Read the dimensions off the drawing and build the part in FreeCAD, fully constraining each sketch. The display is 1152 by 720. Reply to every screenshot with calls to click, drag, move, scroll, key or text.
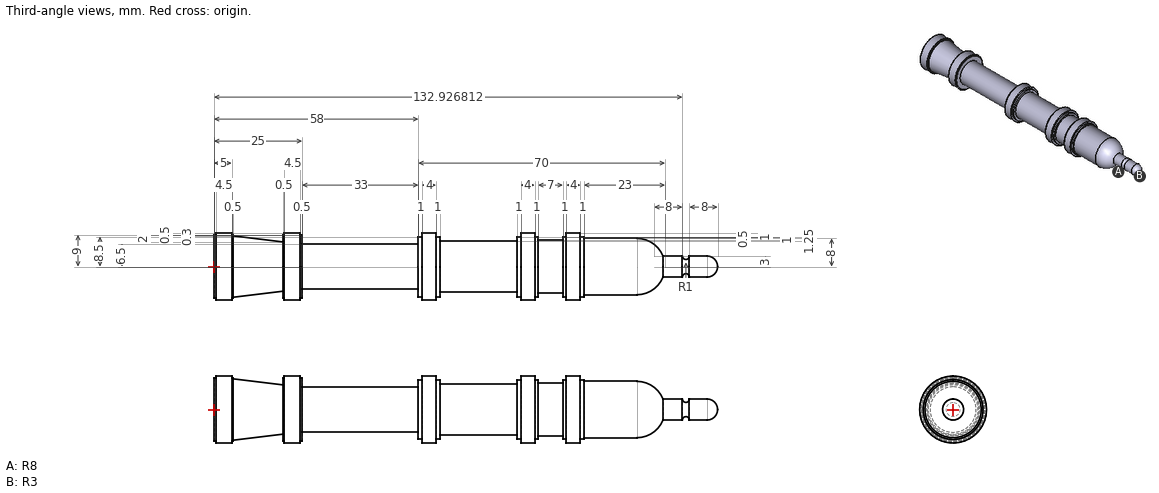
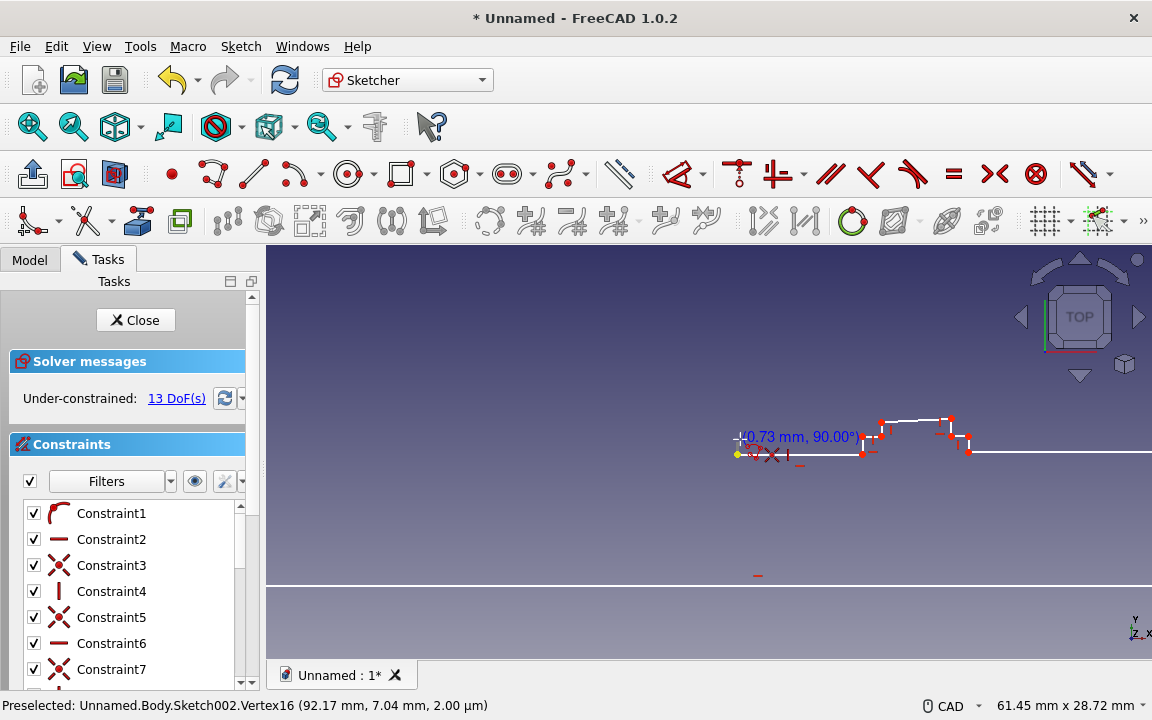
click(738, 436)
click(722, 436)
click(722, 419)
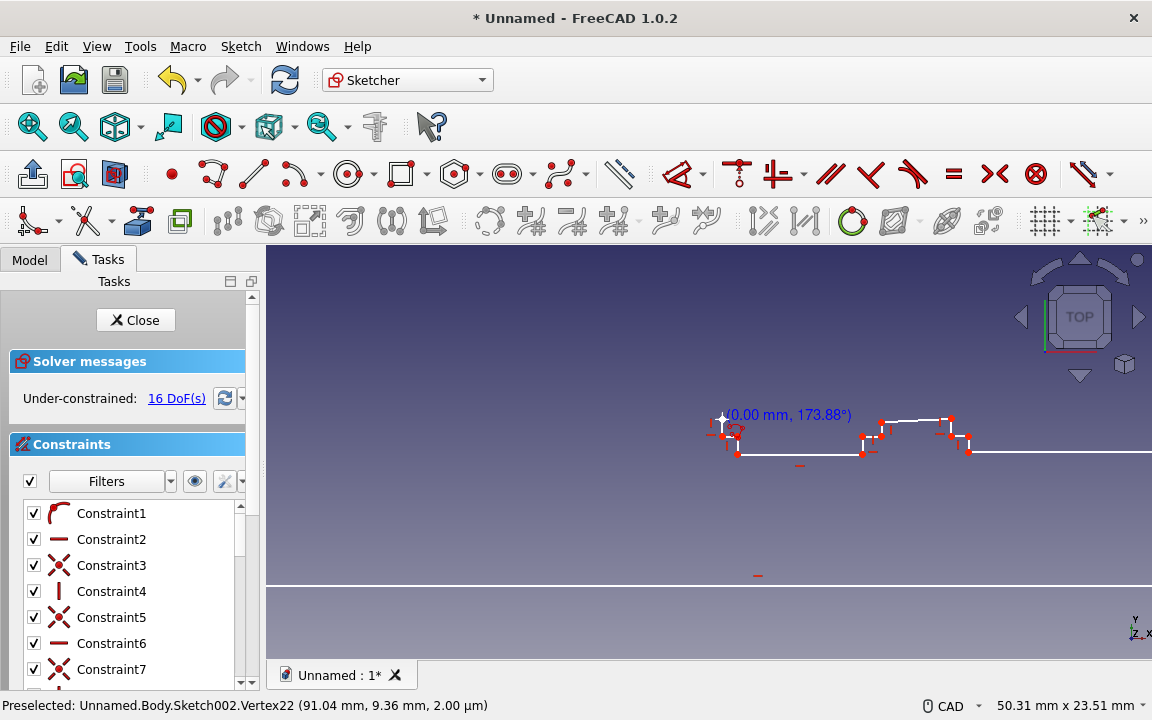
scroll(740, 439, down, 8)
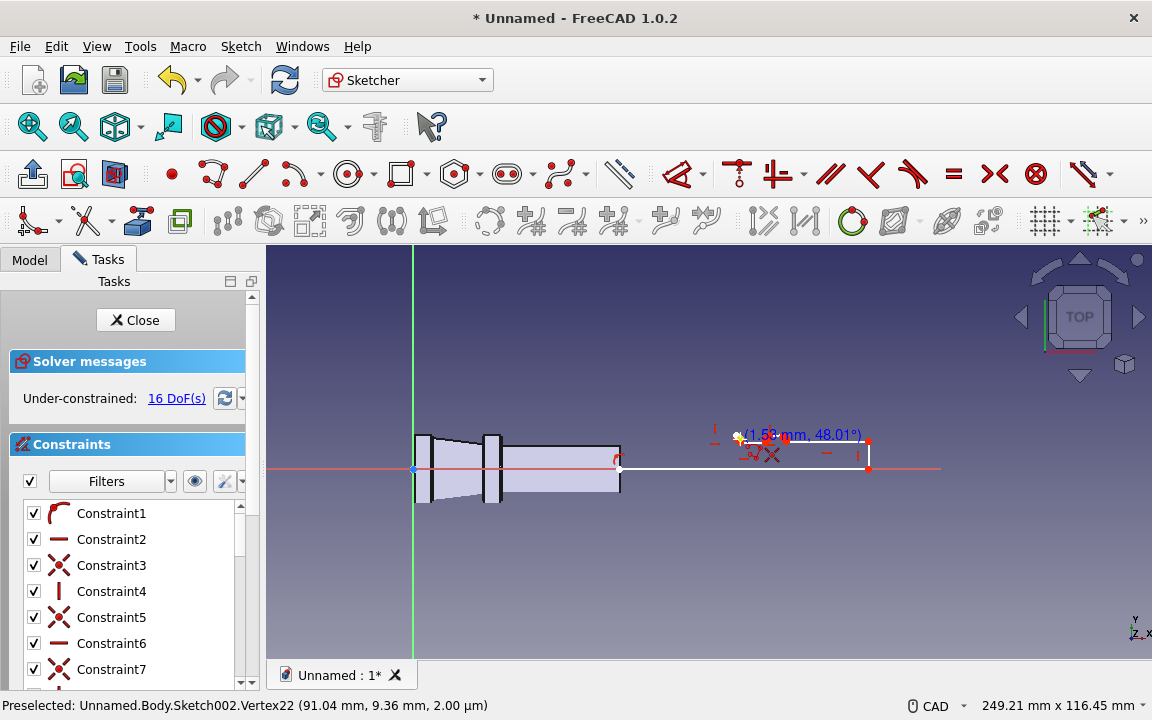
click(723, 435)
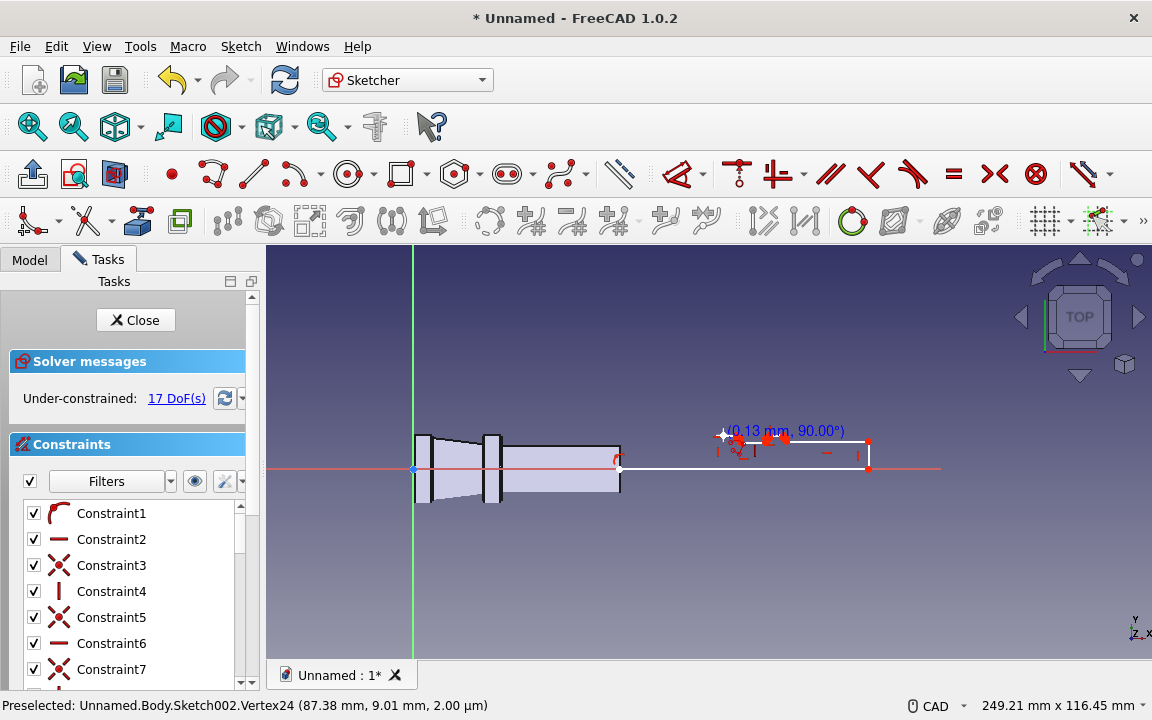
scroll(723, 439, up, 8)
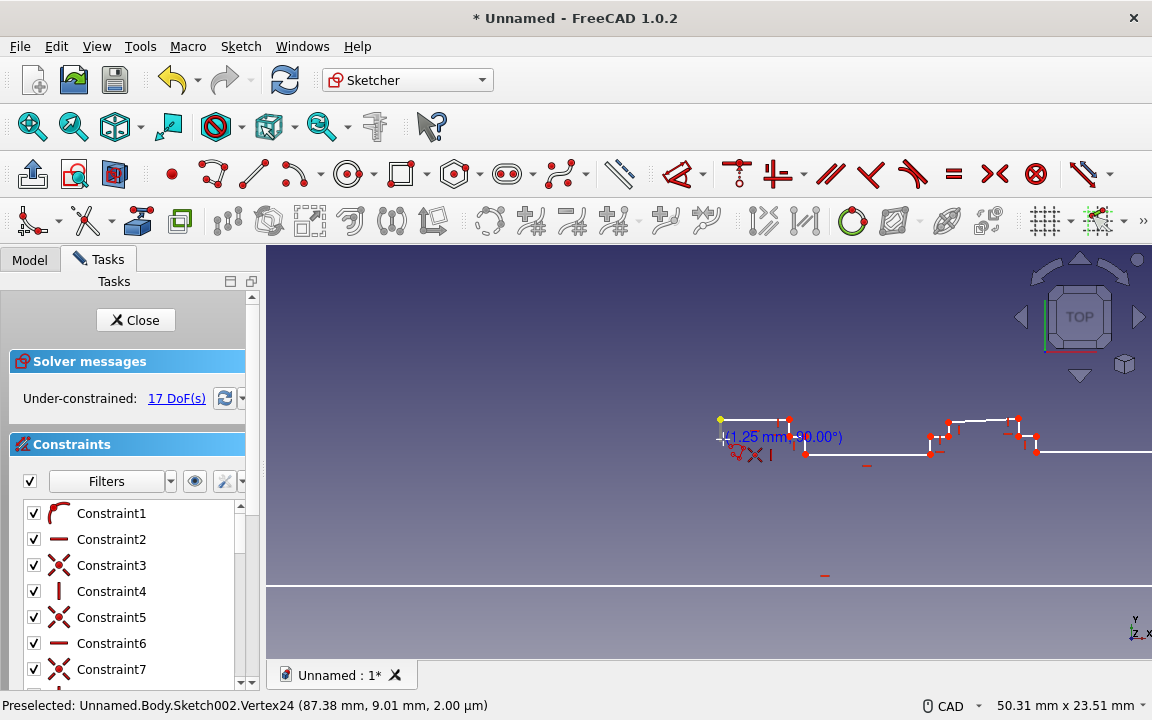
click(721, 436)
click(702, 436)
click(702, 458)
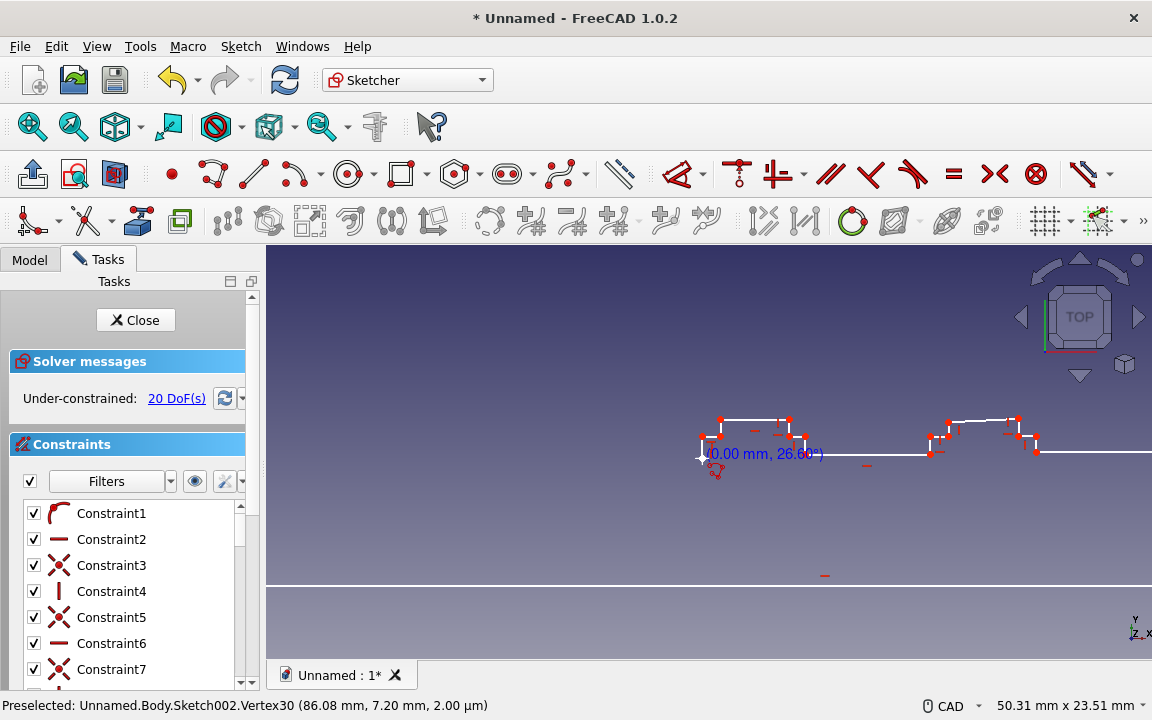
scroll(723, 439, down, 8)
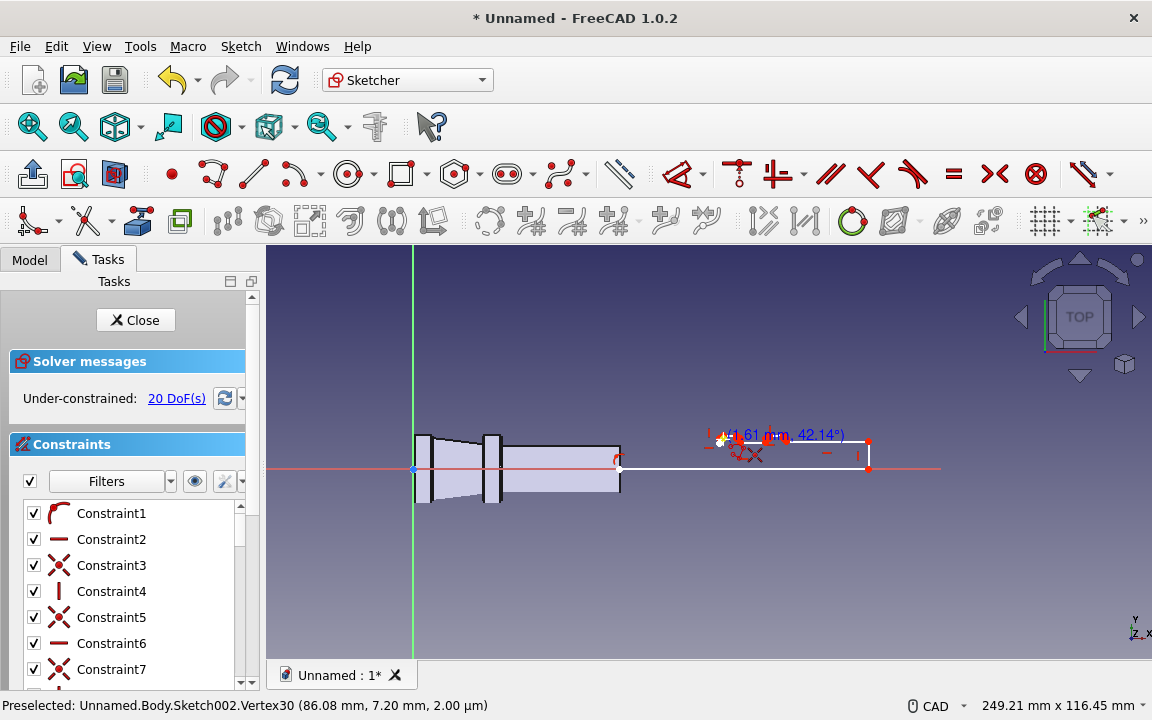
click(641, 443)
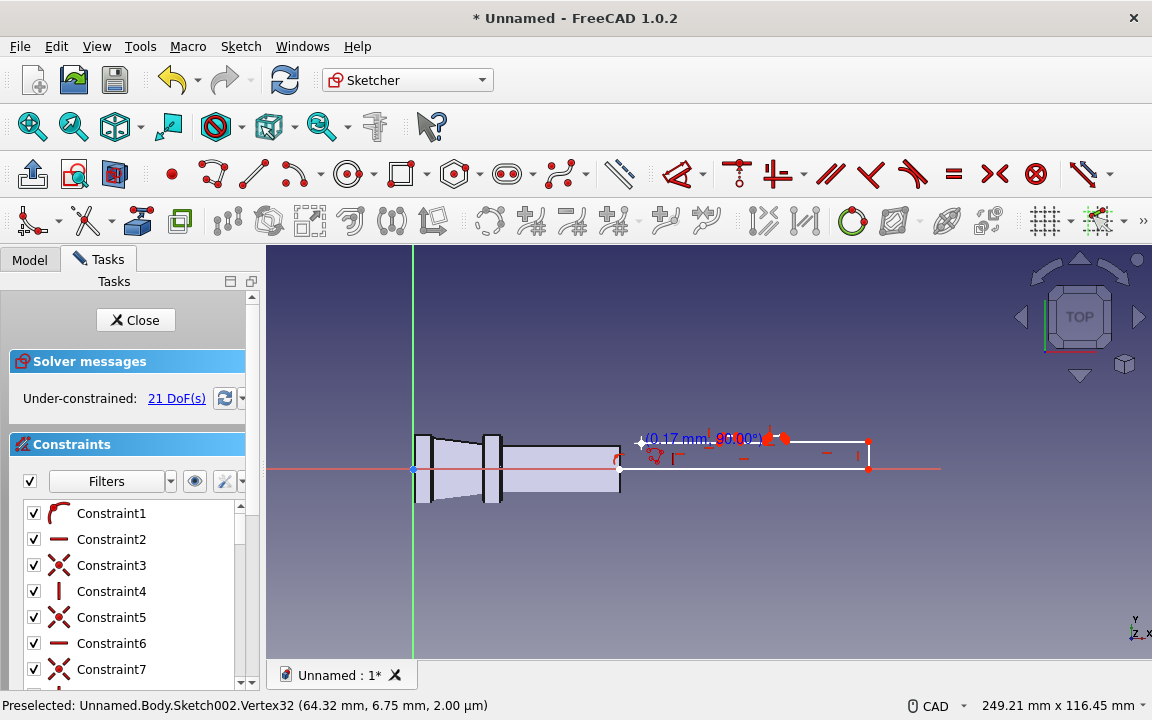
scroll(641, 439, up, 7)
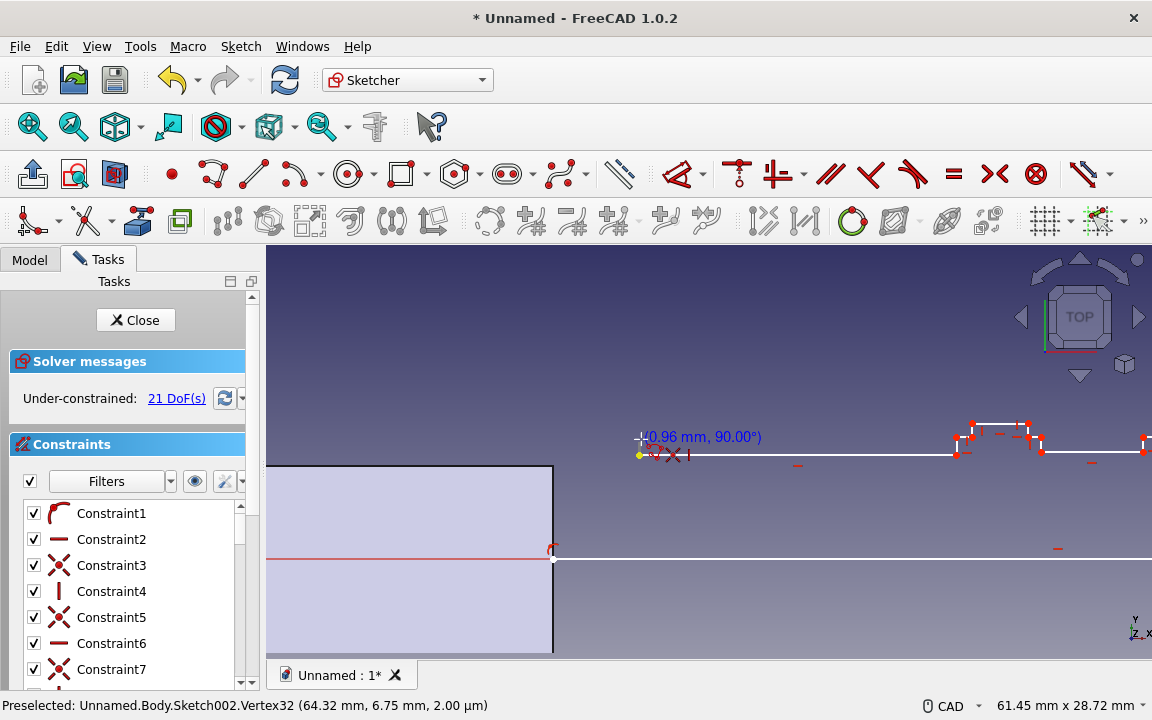
click(640, 437)
click(625, 437)
click(625, 422)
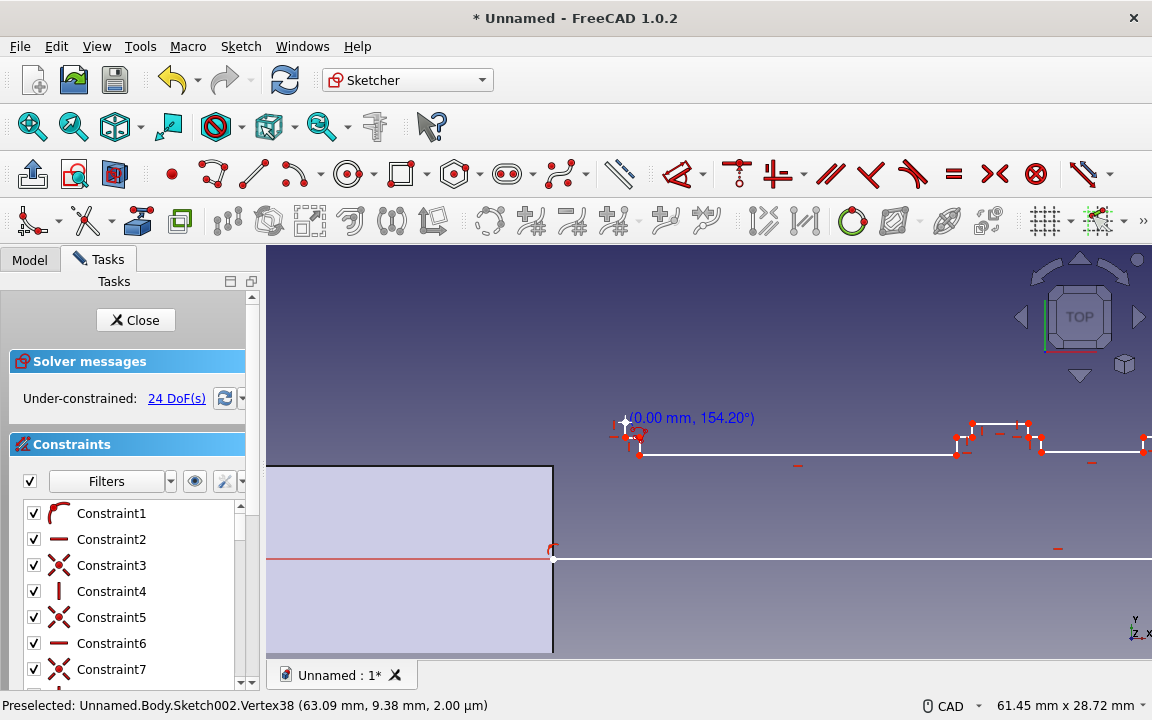
scroll(641, 439, down, 7)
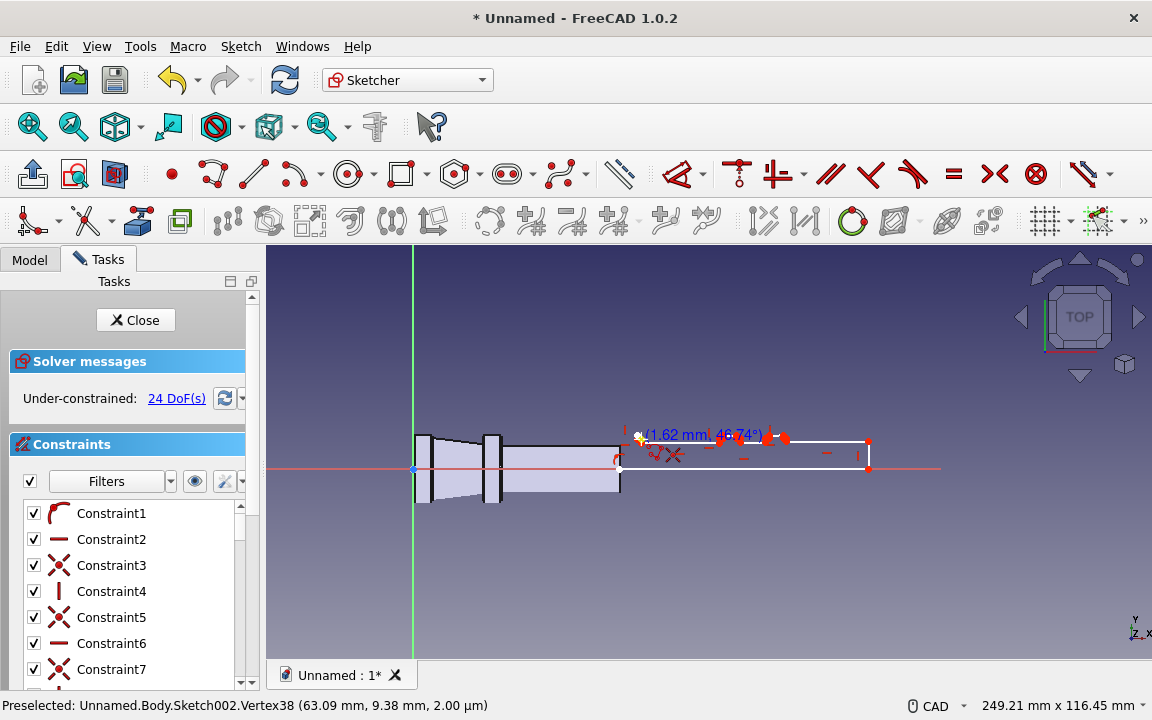
click(623, 435)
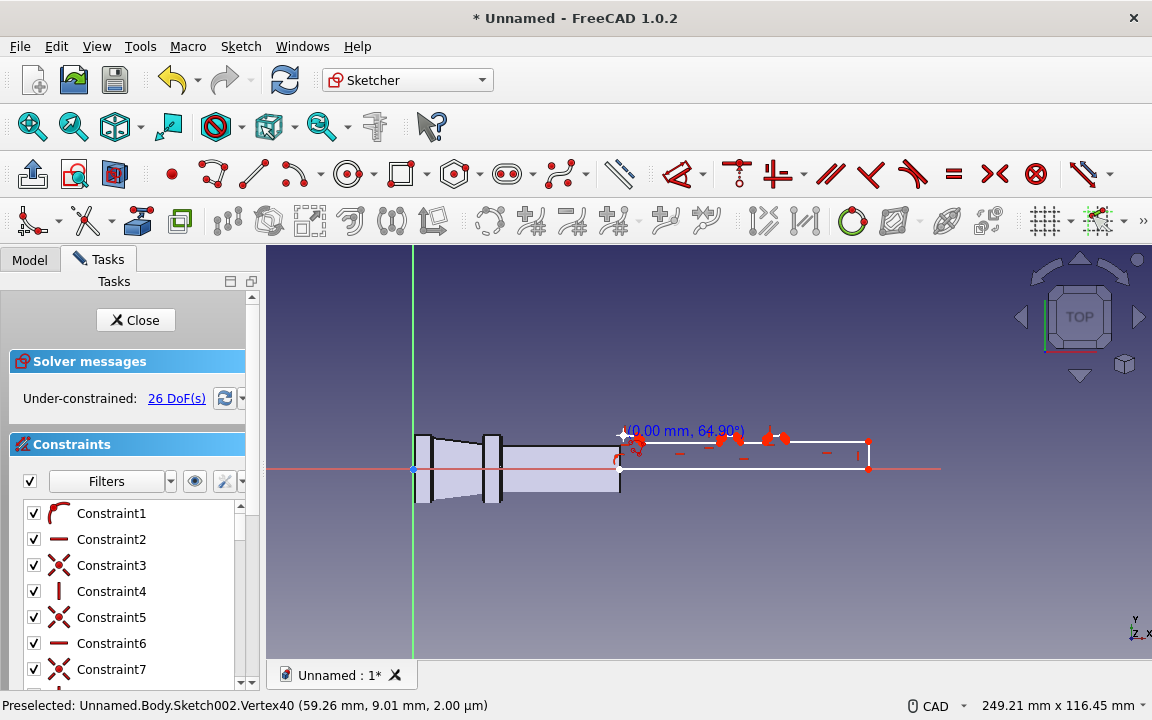
scroll(623, 439, up, 8)